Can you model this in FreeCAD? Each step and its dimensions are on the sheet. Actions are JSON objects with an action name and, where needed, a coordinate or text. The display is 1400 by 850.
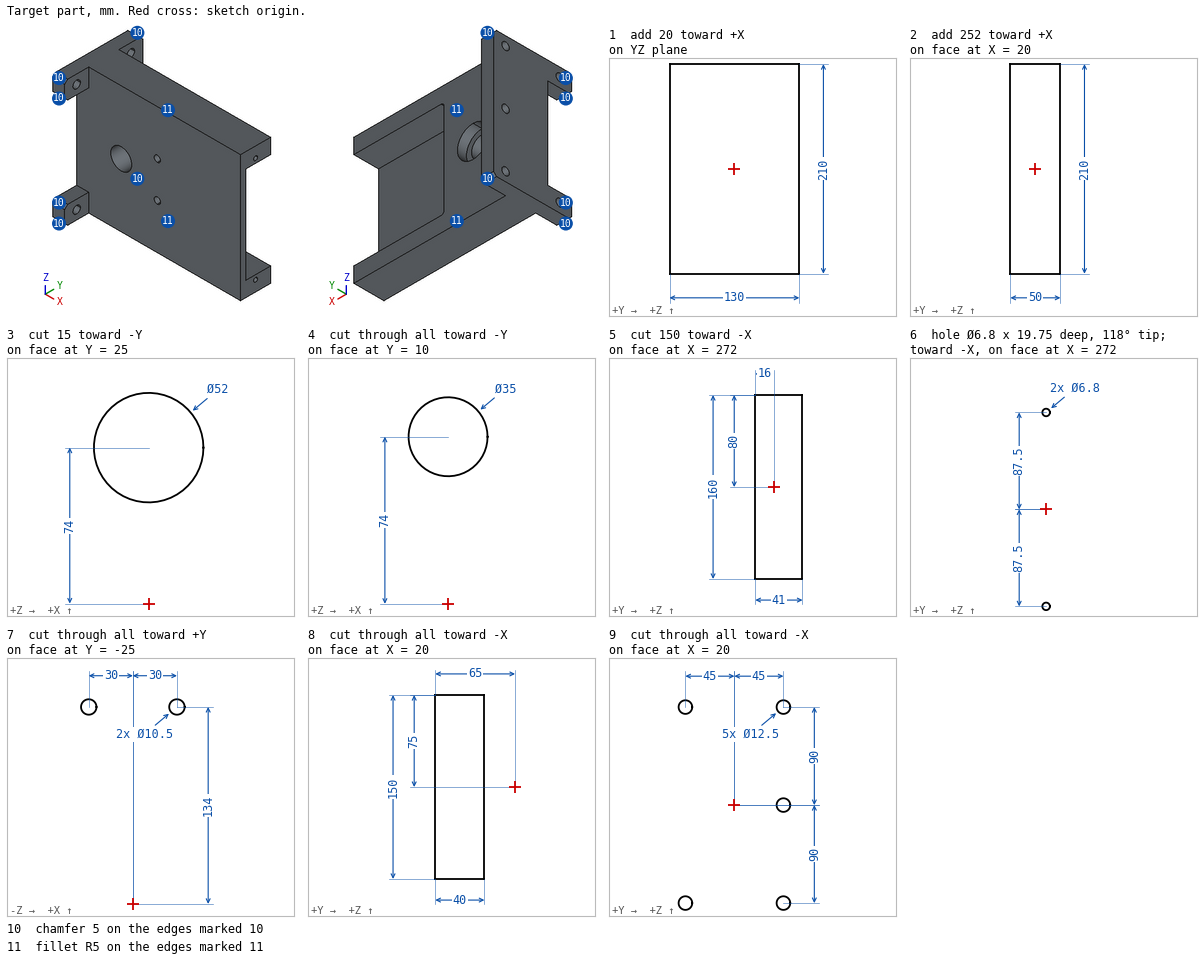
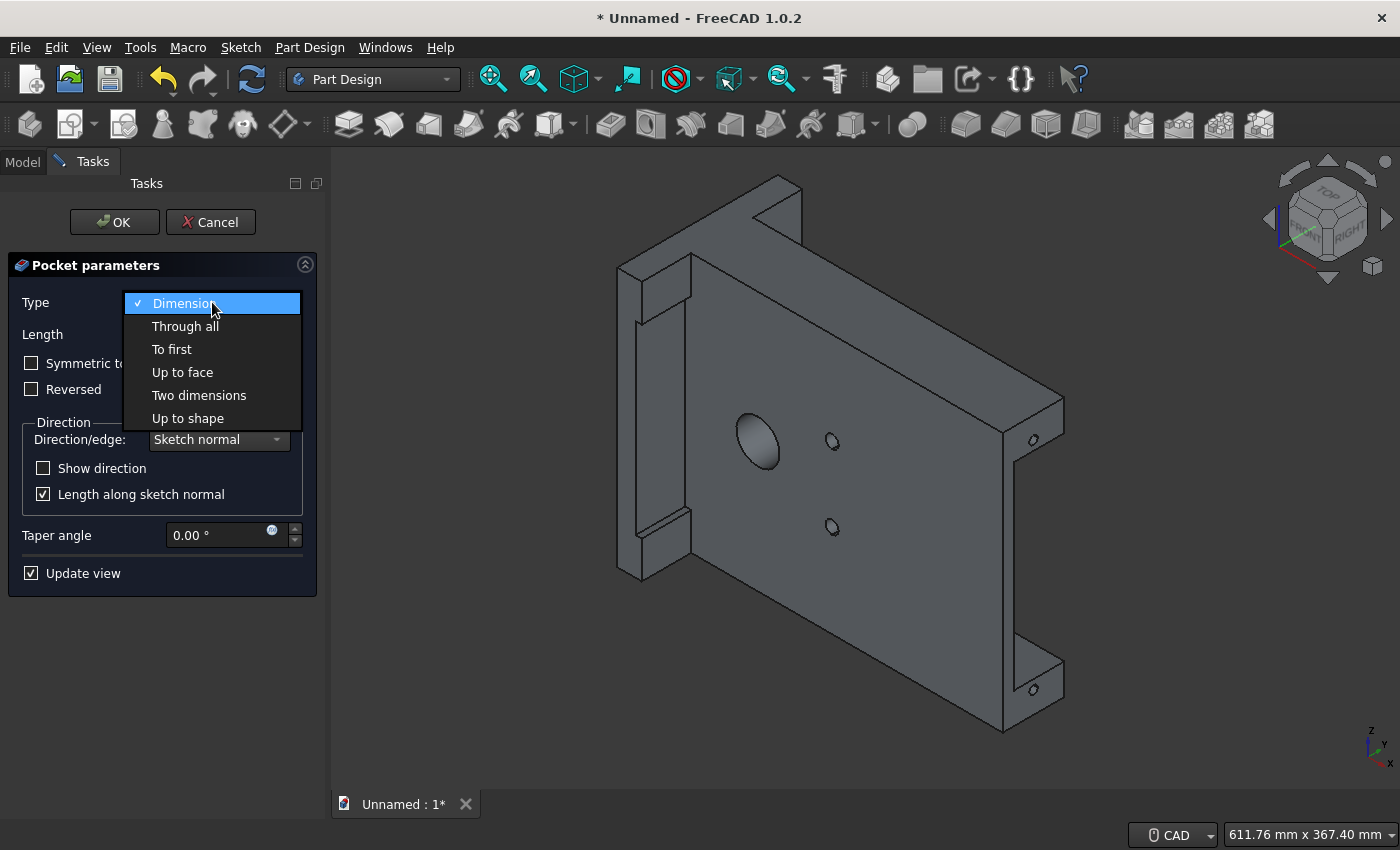
{"action": "left_click", "coordinate": [212, 326]}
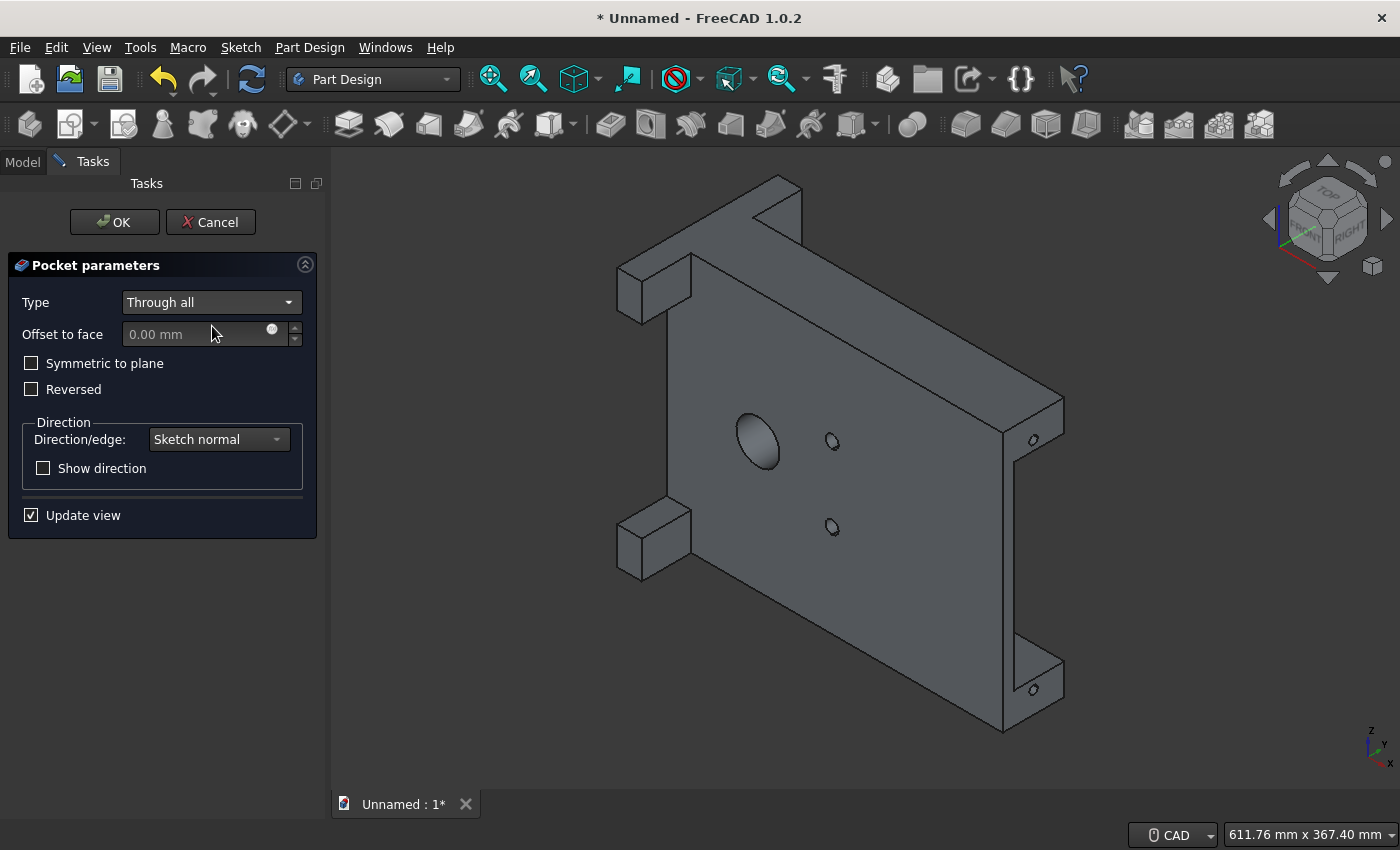
{"action": "left_click", "coordinate": [115, 222]}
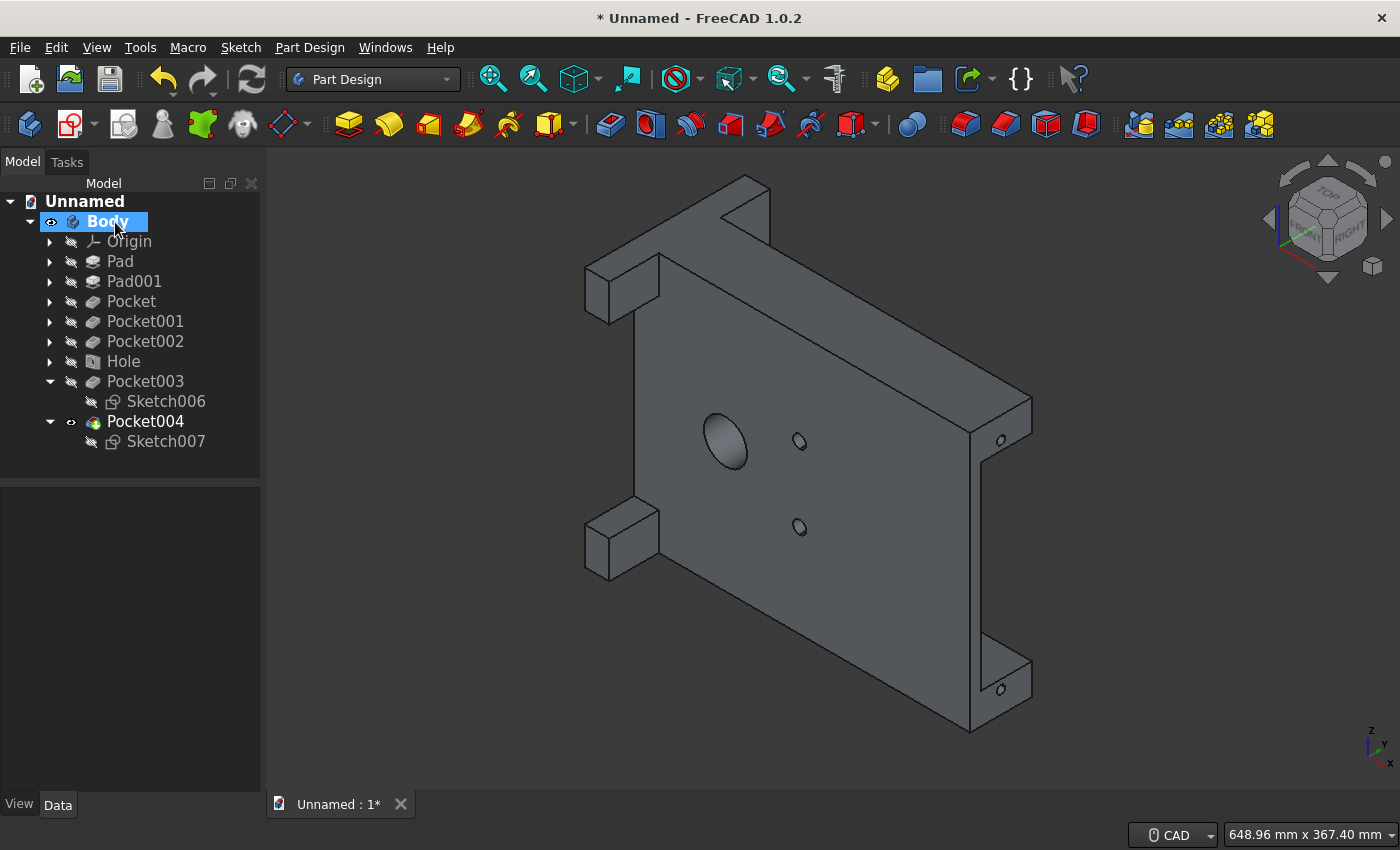
{"action": "key", "text": "3"}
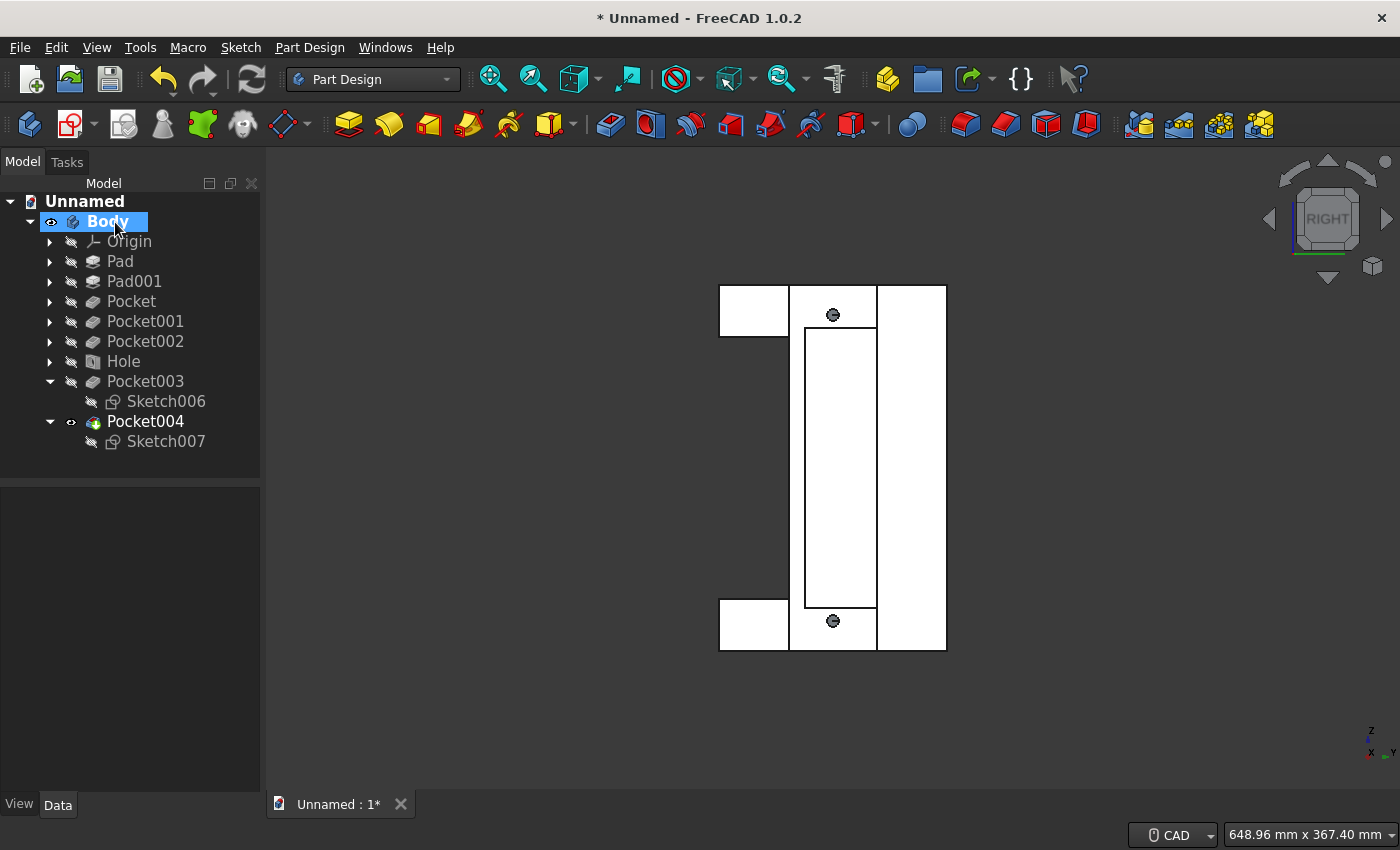
{"action": "left_click", "coordinate": [912, 415]}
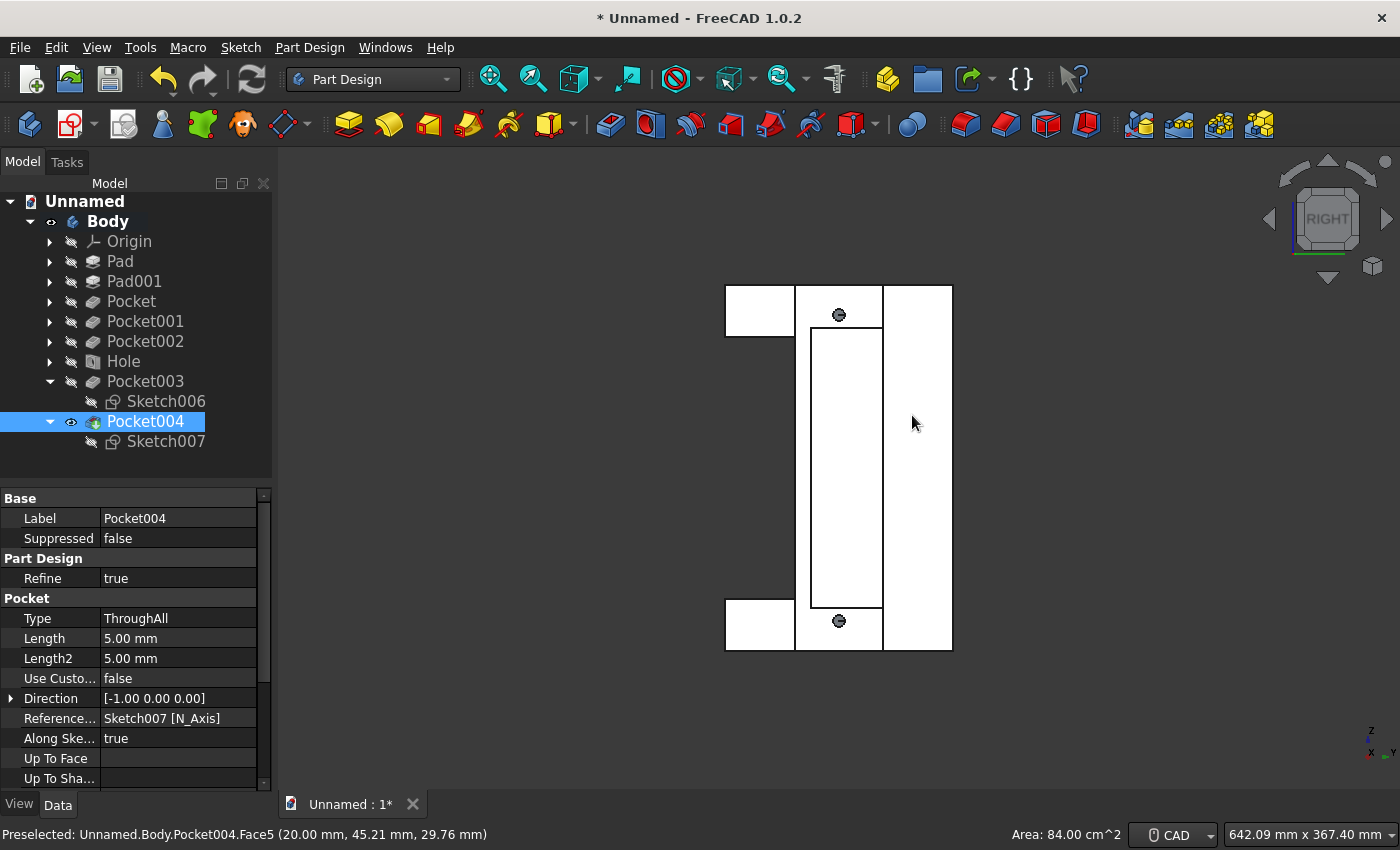
{"action": "left_click", "coordinate": [70, 124]}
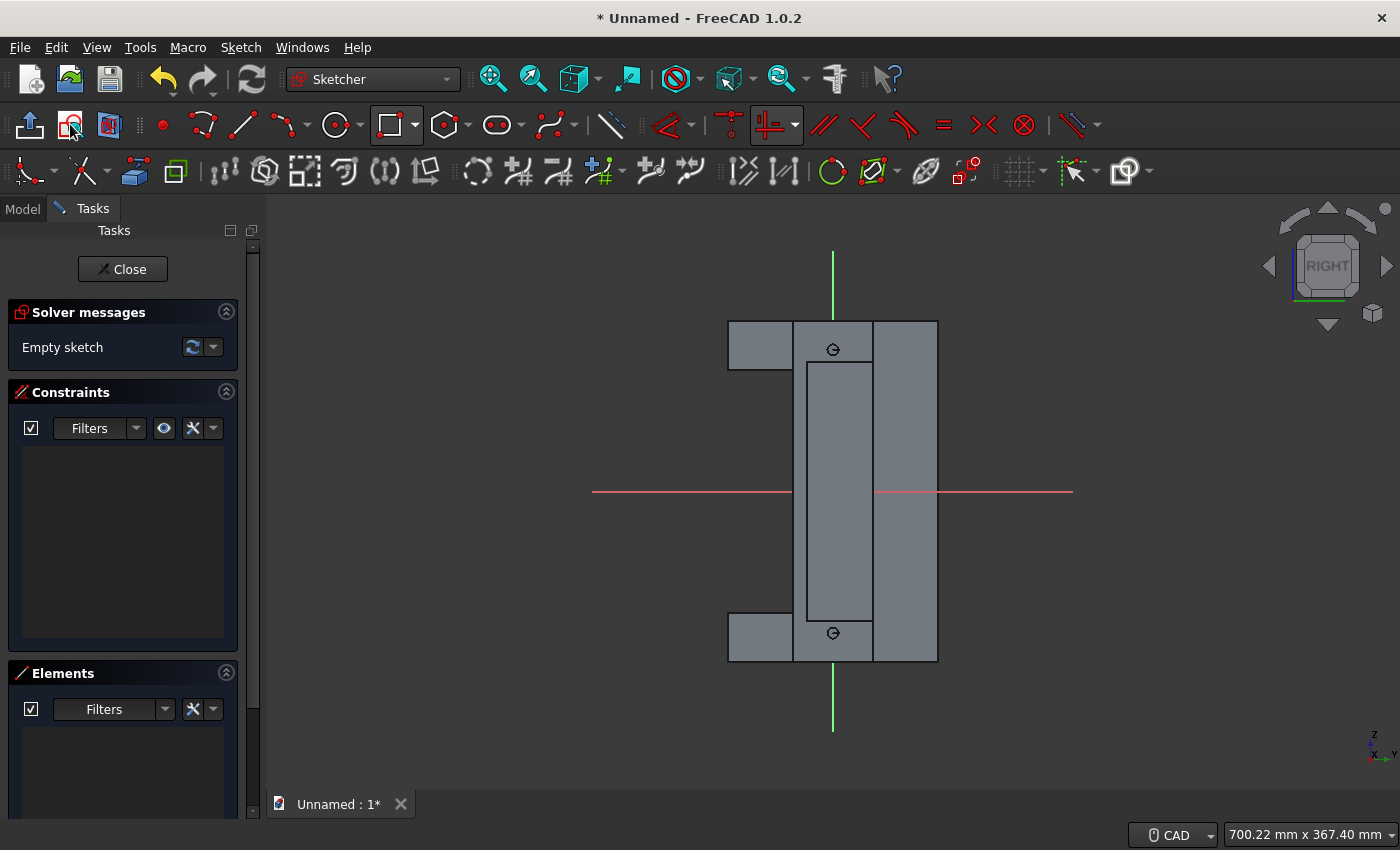
{"action": "left_click", "coordinate": [110, 126]}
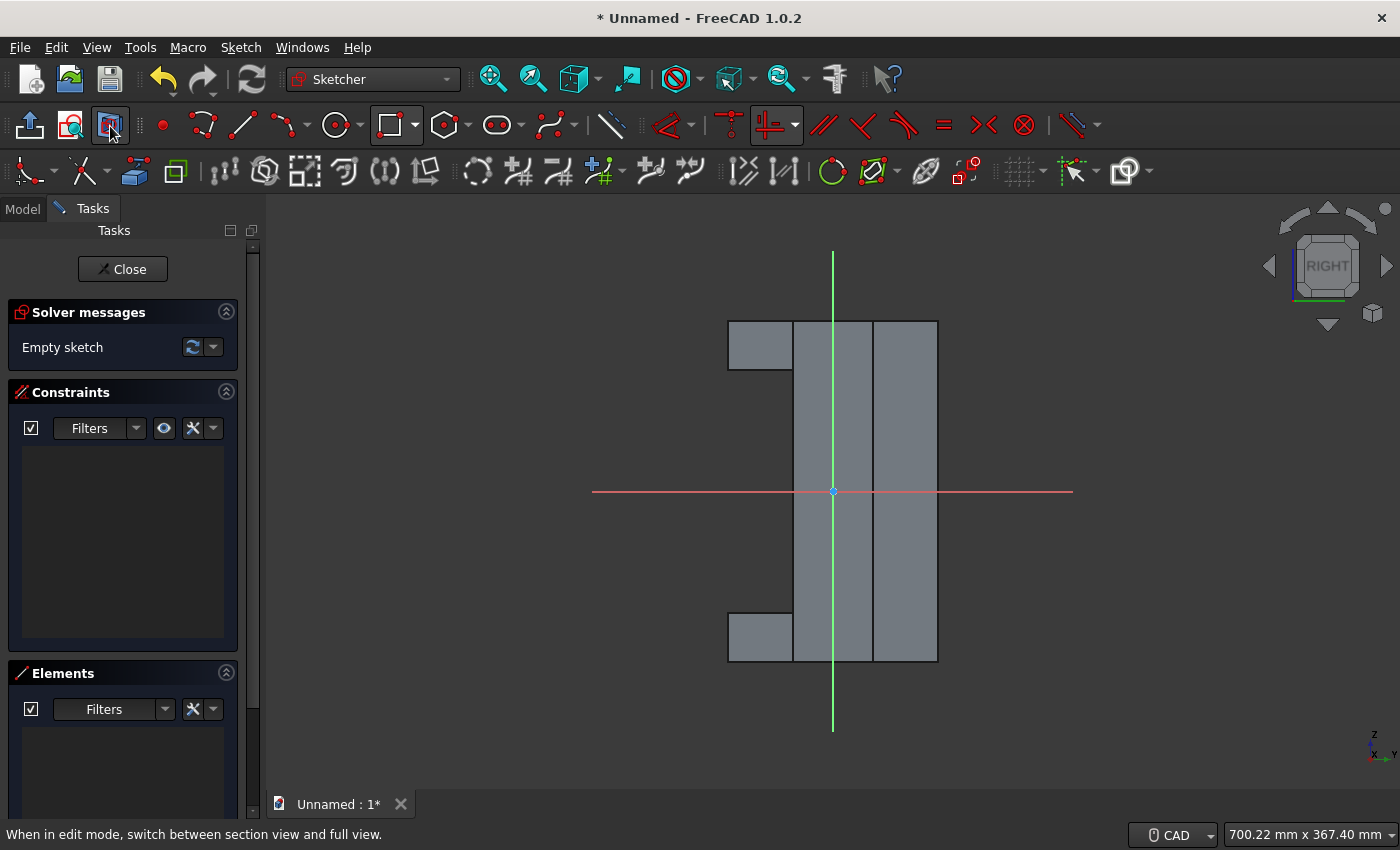
{"action": "left_click", "coordinate": [336, 126]}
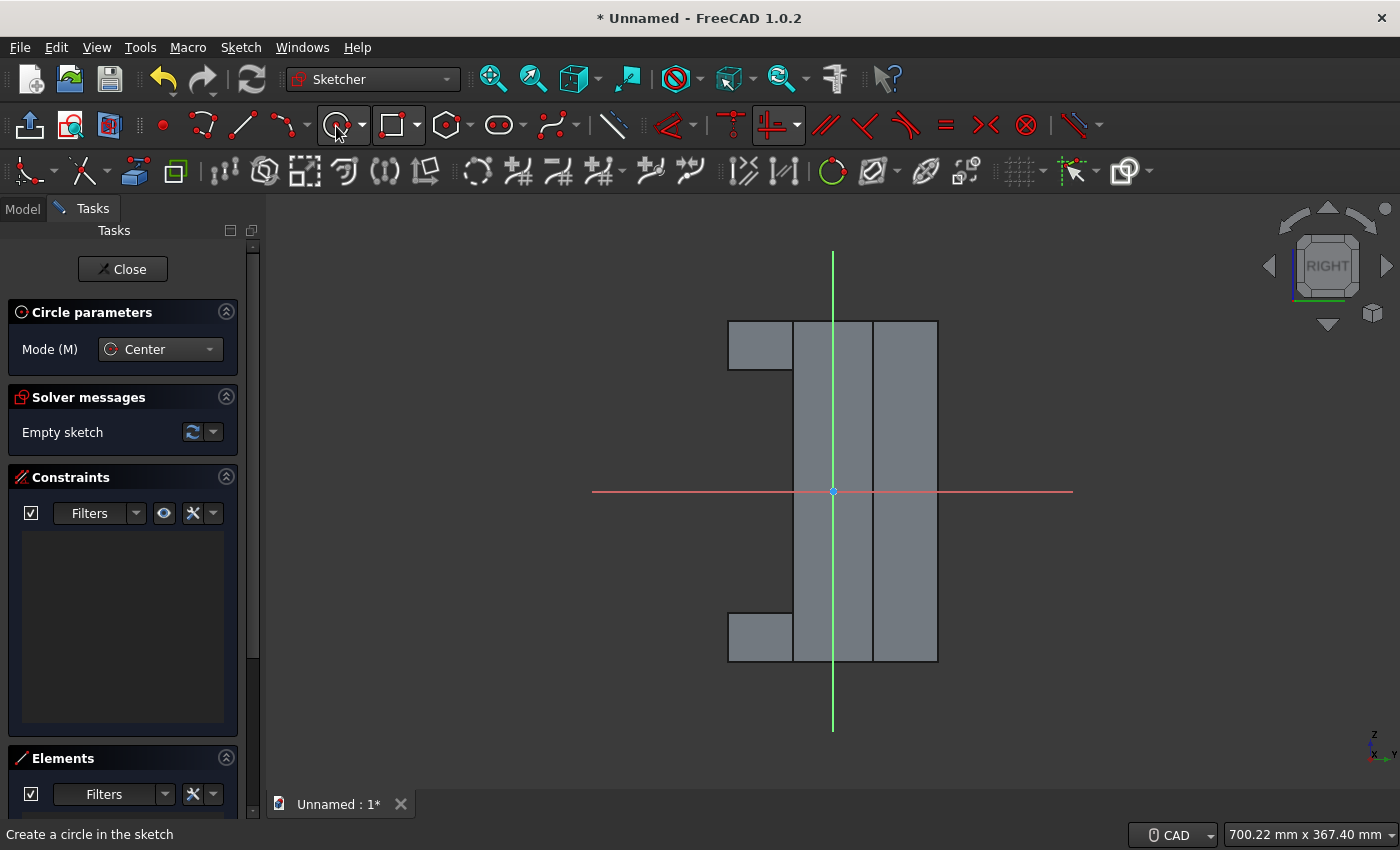
{"action": "scroll", "coordinate": [906, 346], "scroll_direction": "up", "scroll_amount": 5}